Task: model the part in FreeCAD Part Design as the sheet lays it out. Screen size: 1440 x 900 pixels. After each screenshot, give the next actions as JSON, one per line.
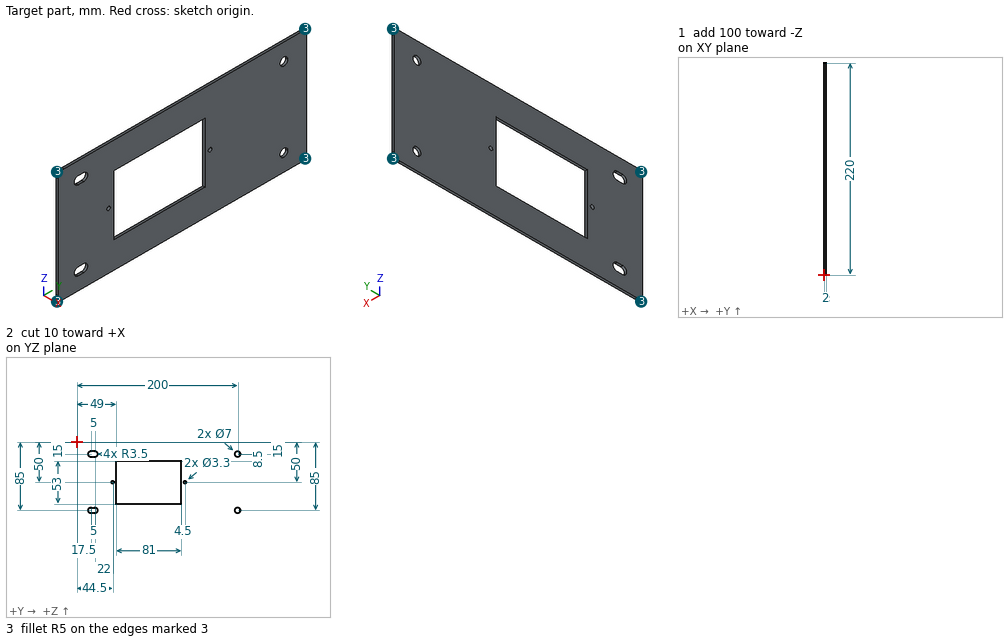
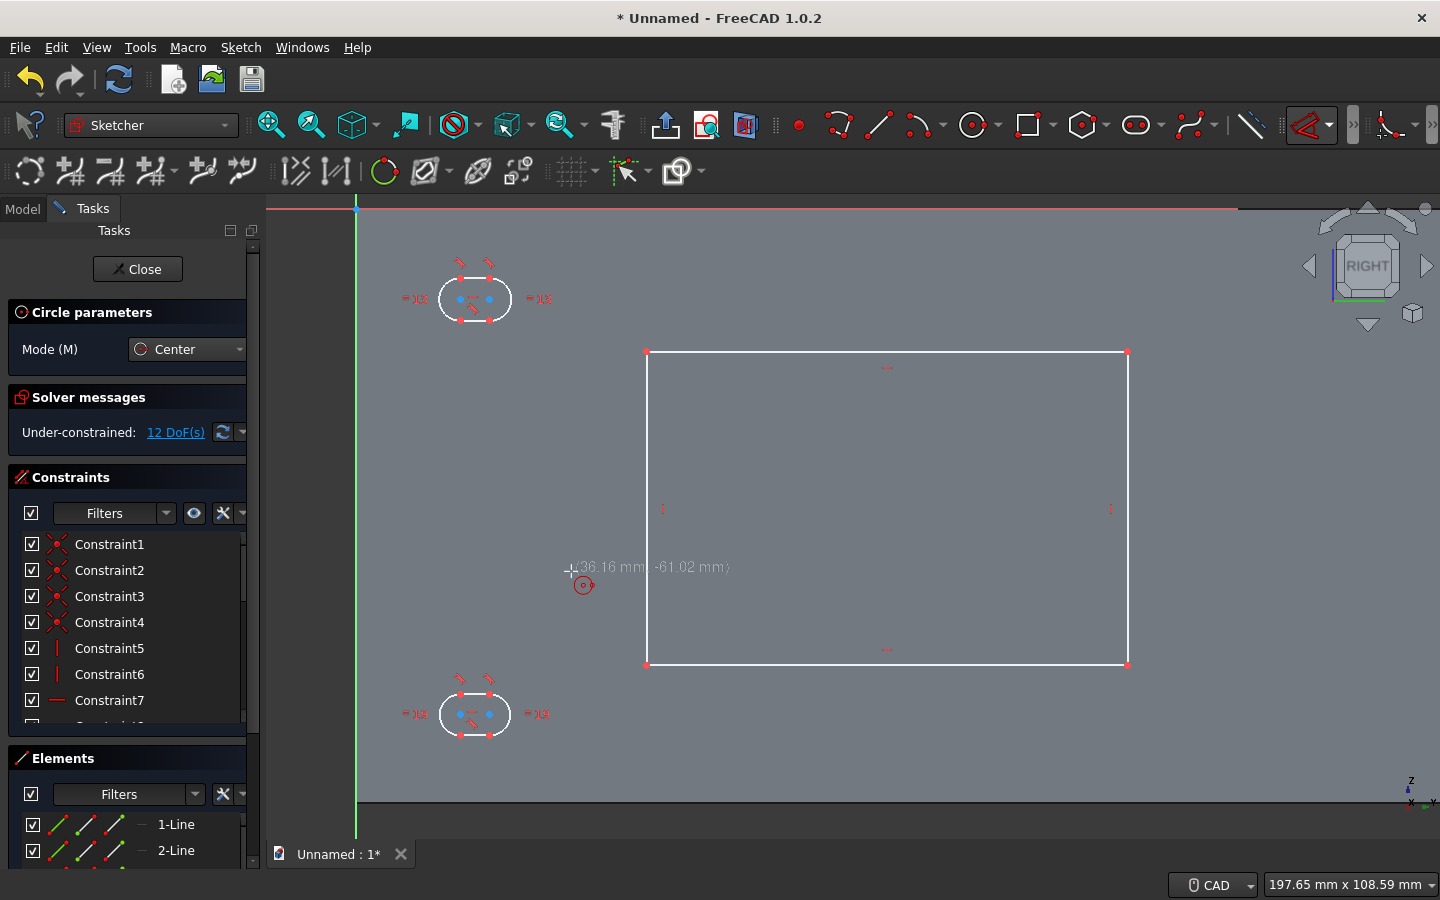
{"action": "left_click", "coordinate": [598, 536]}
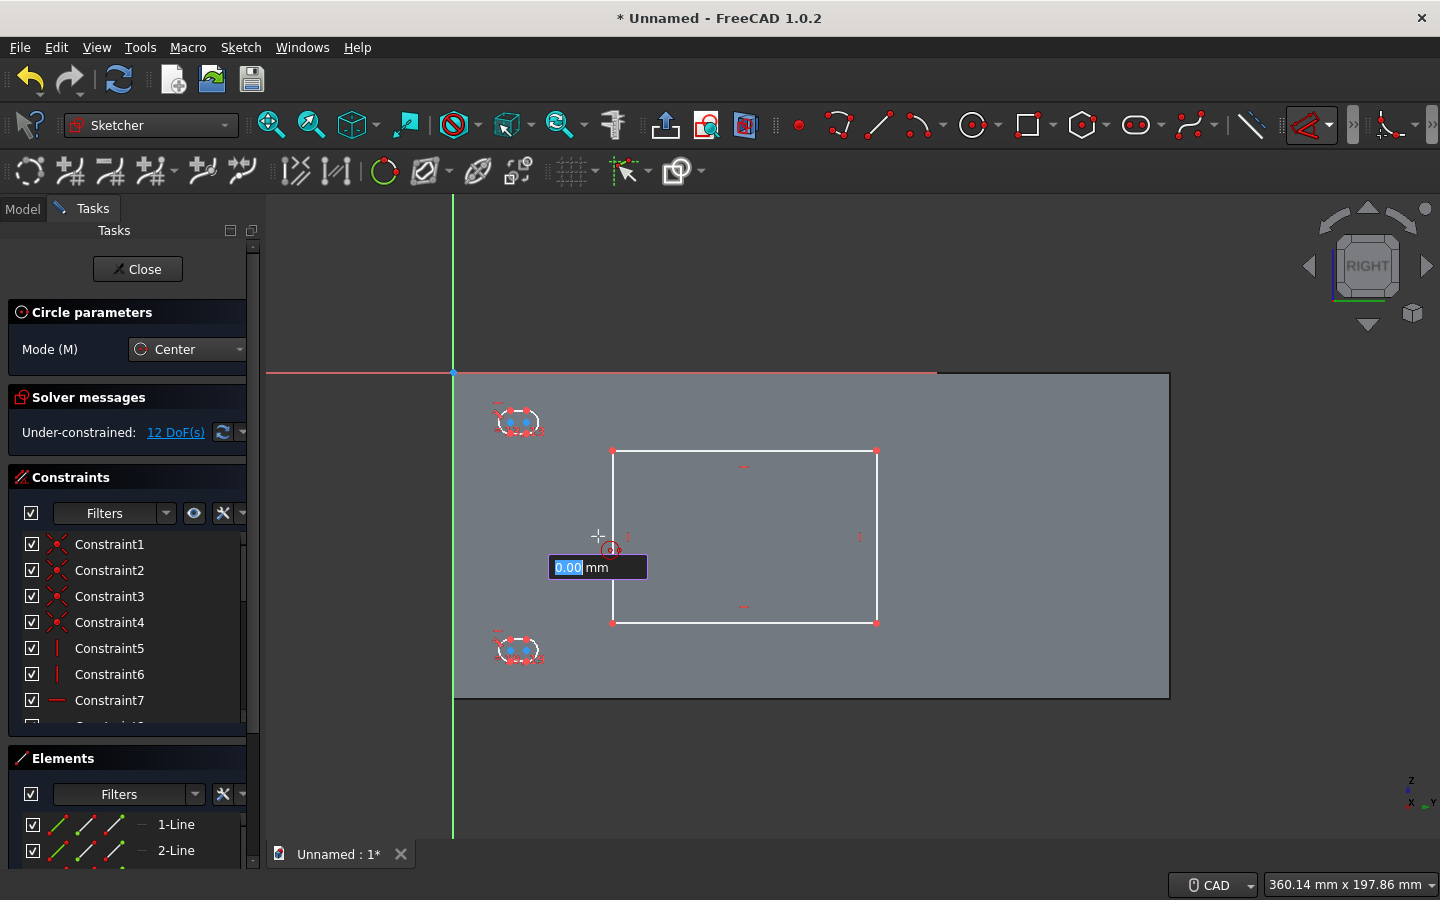
{"action": "scroll", "coordinate": [595, 532], "scroll_direction": "up", "scroll_amount": 6}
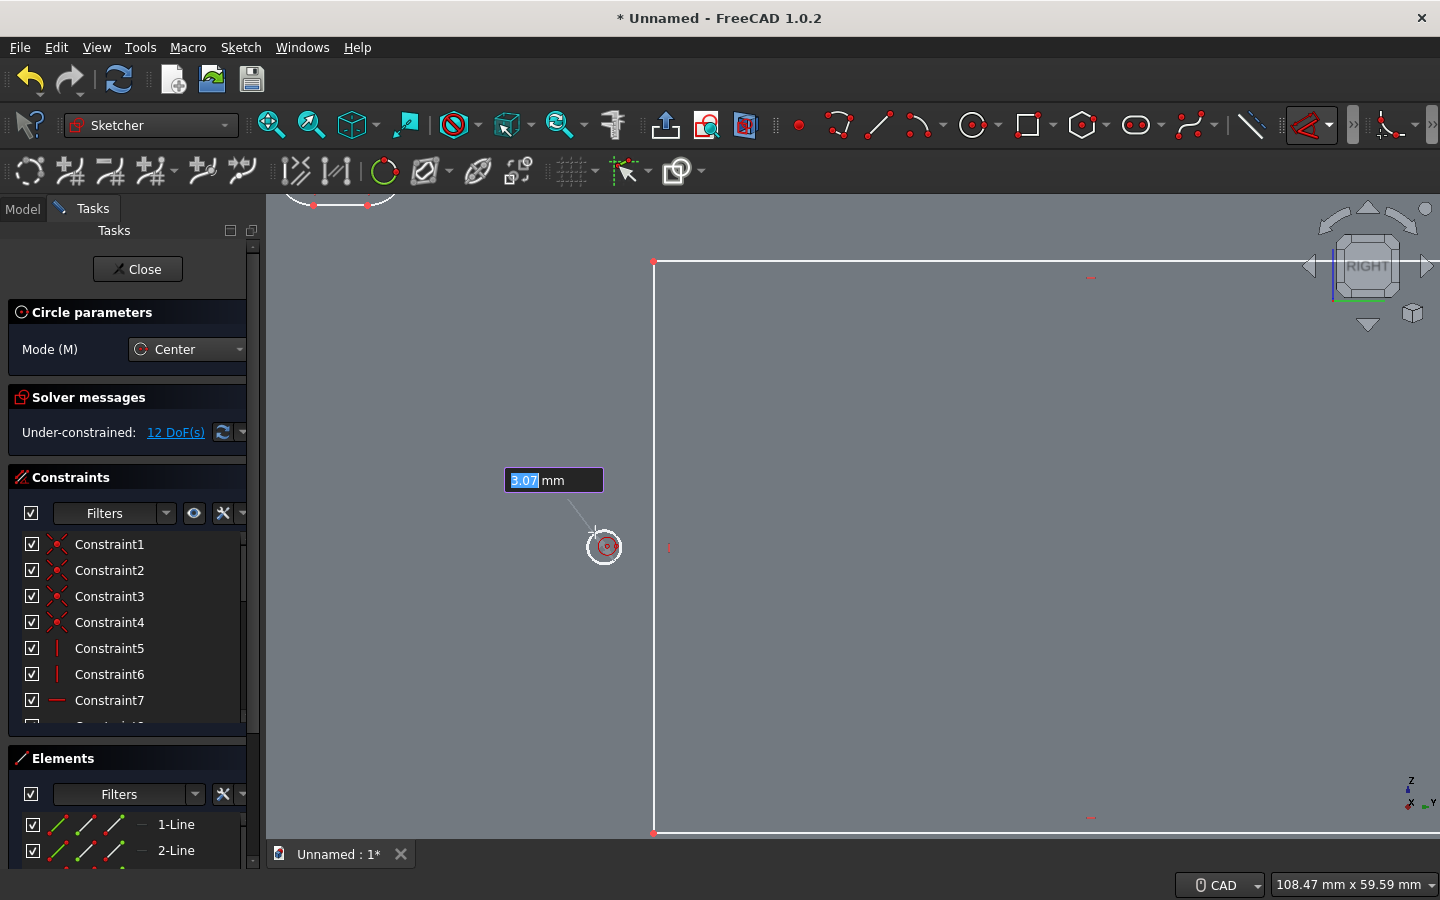
{"action": "left_click", "coordinate": [593, 531]}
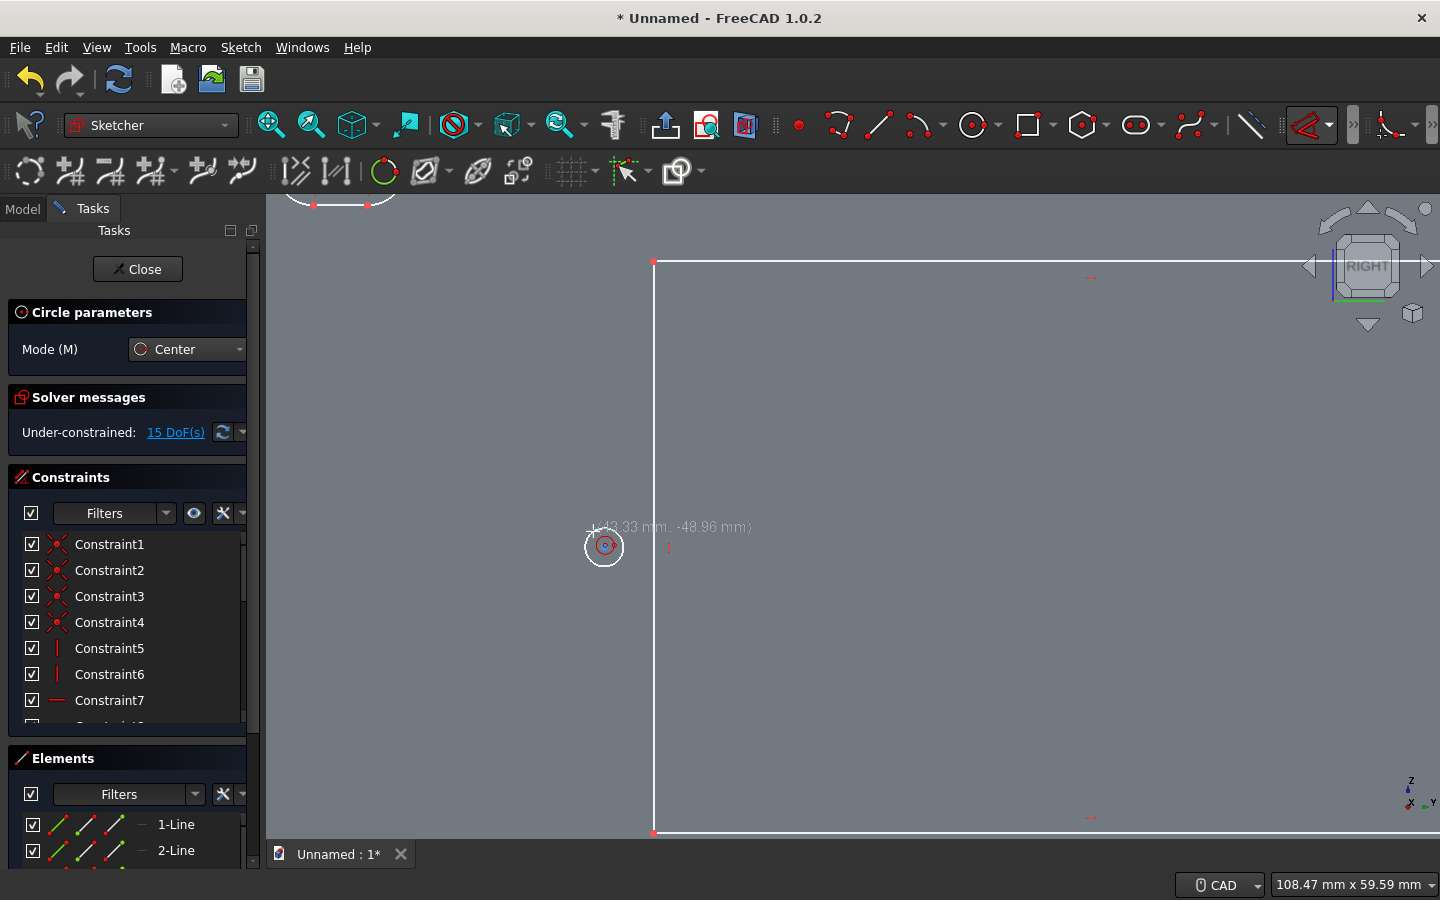
{"action": "scroll", "coordinate": [595, 532], "scroll_direction": "down", "scroll_amount": 6}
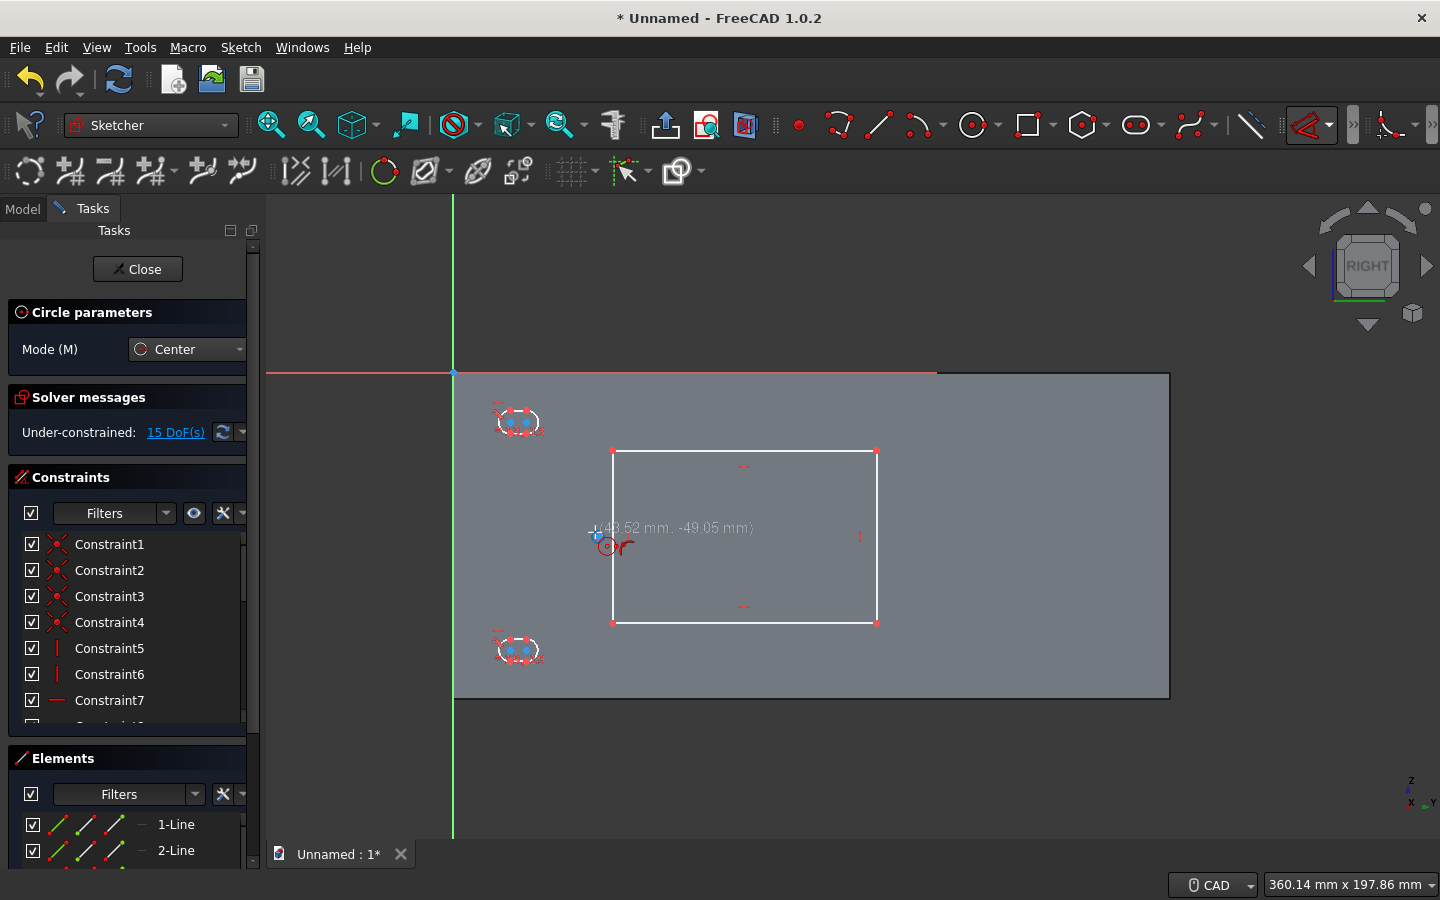
{"action": "scroll", "coordinate": [892, 536], "scroll_direction": "up", "scroll_amount": 8}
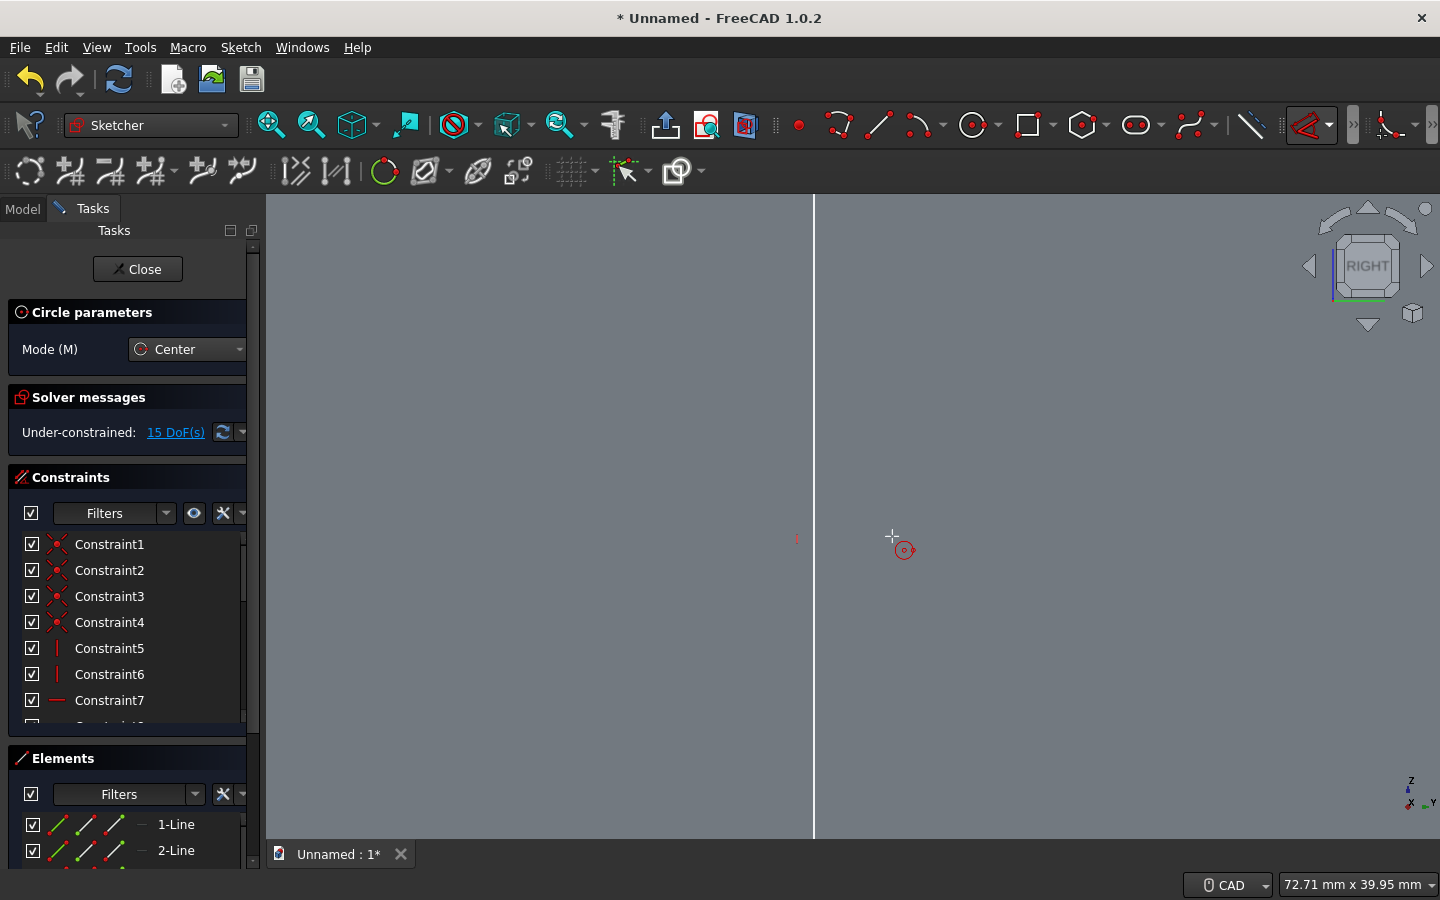
{"action": "scroll", "coordinate": [892, 536], "scroll_direction": "down", "scroll_amount": 8}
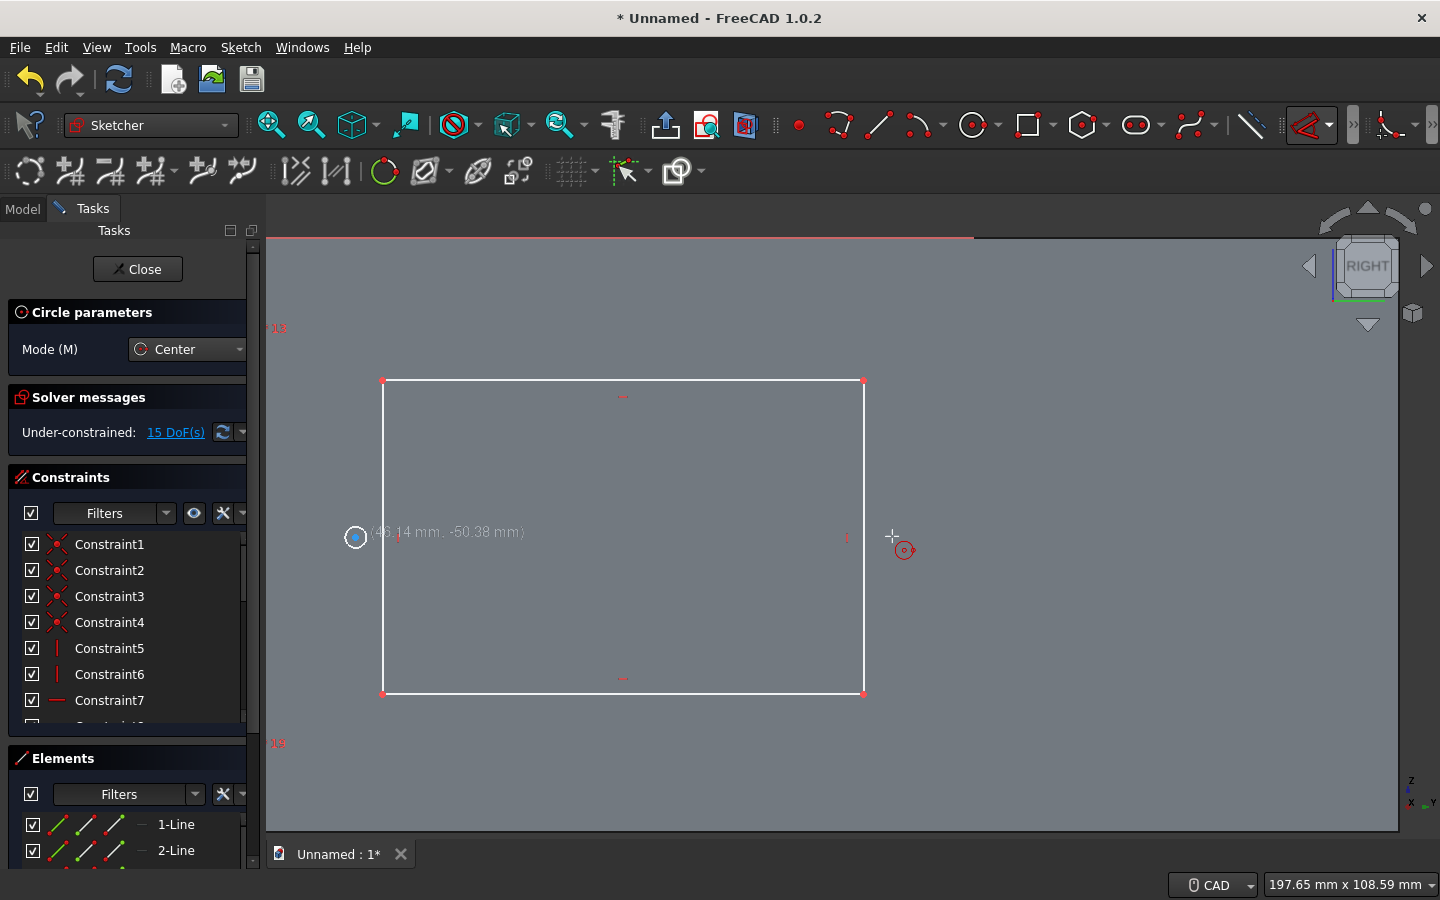
{"action": "left_click", "coordinate": [892, 536]}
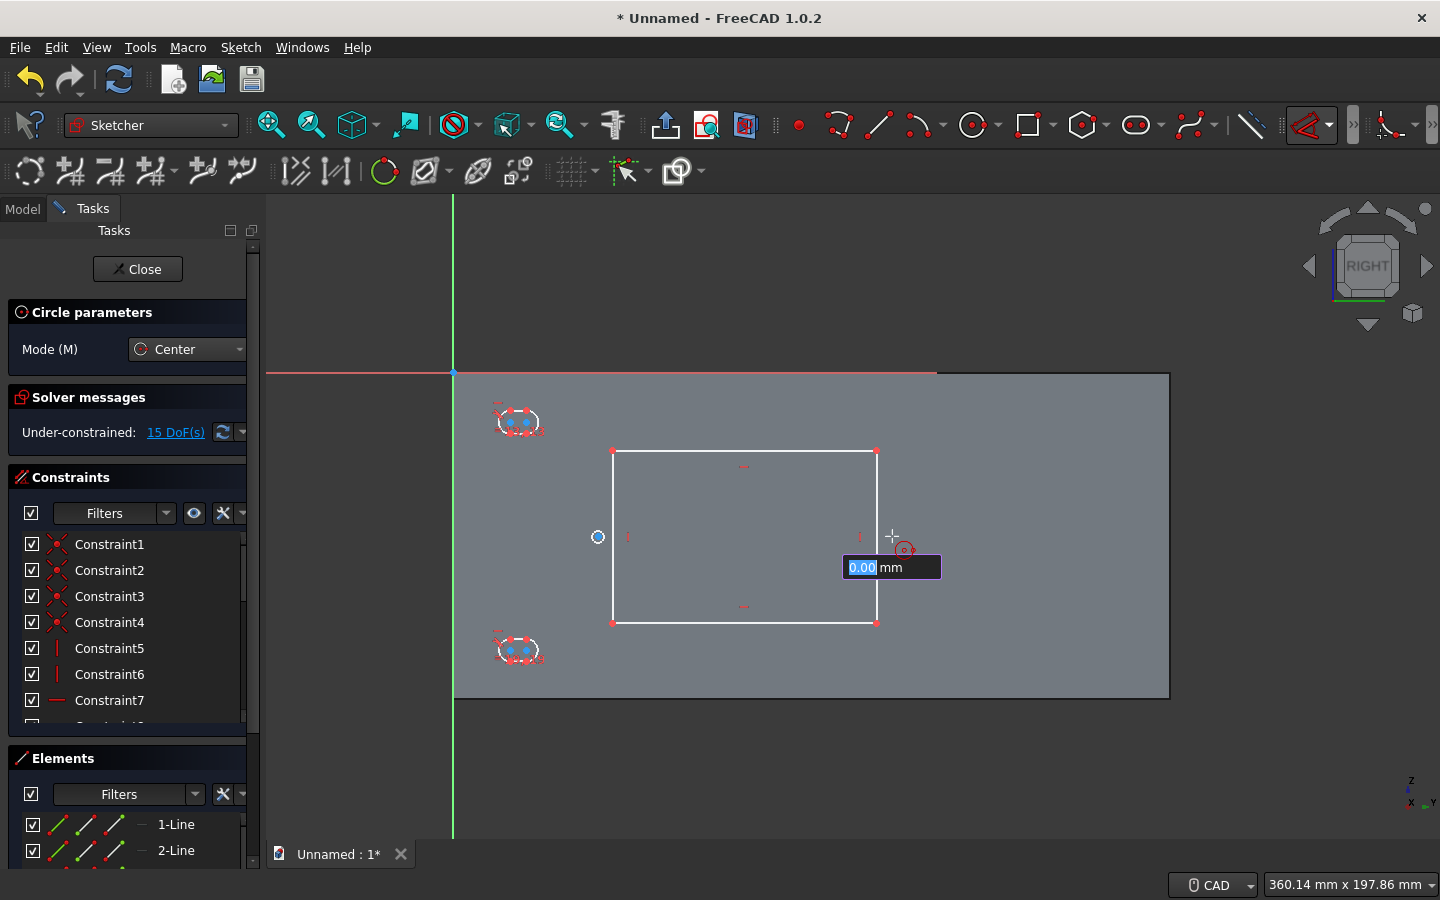
{"action": "scroll", "coordinate": [896, 532], "scroll_direction": "up", "scroll_amount": 6}